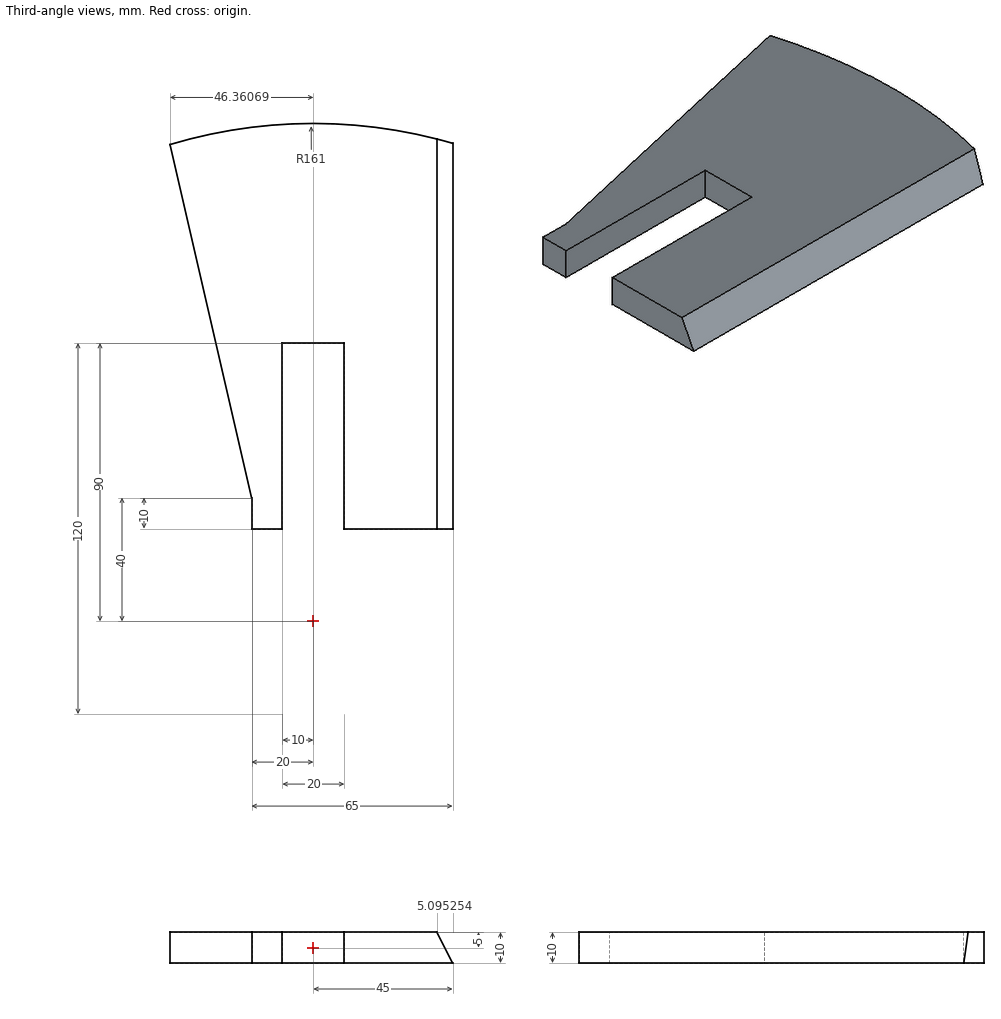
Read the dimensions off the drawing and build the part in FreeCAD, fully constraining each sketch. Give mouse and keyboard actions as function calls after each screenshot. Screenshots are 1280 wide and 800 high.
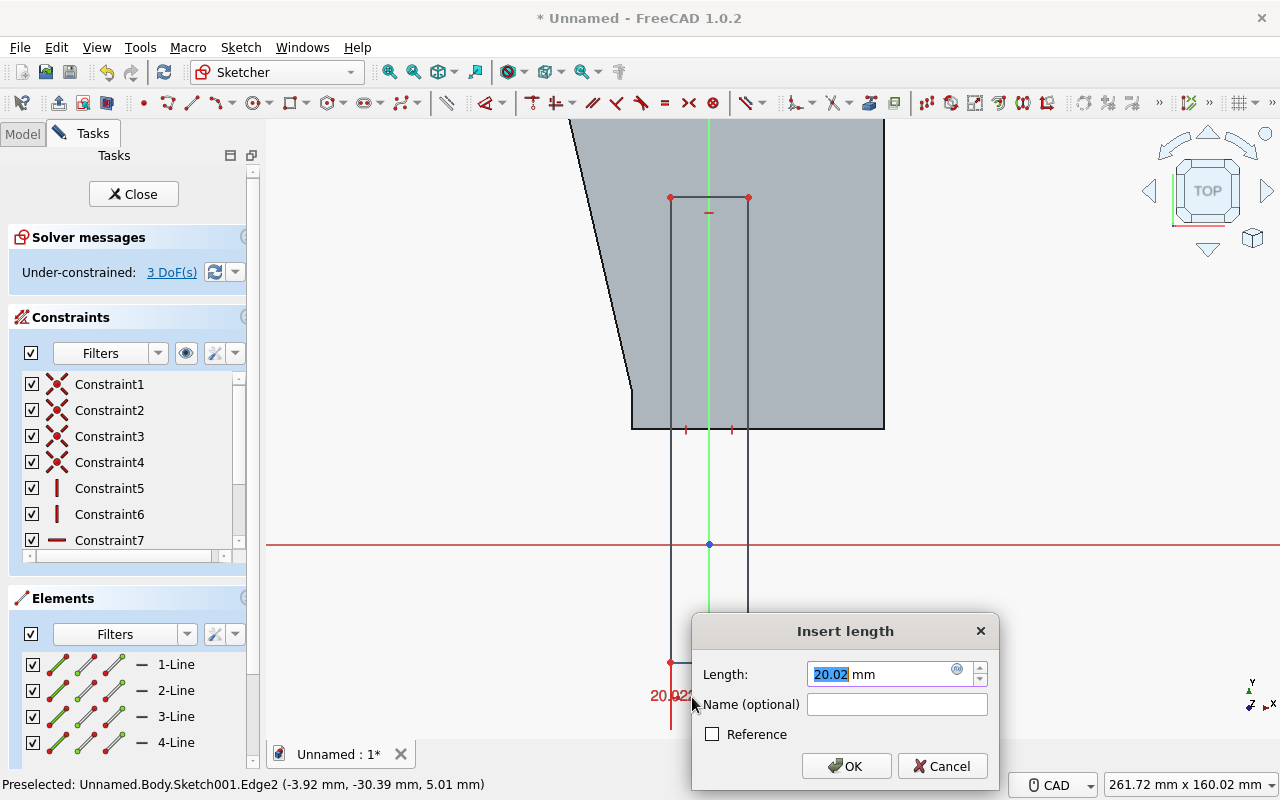
text(20)
key(Return)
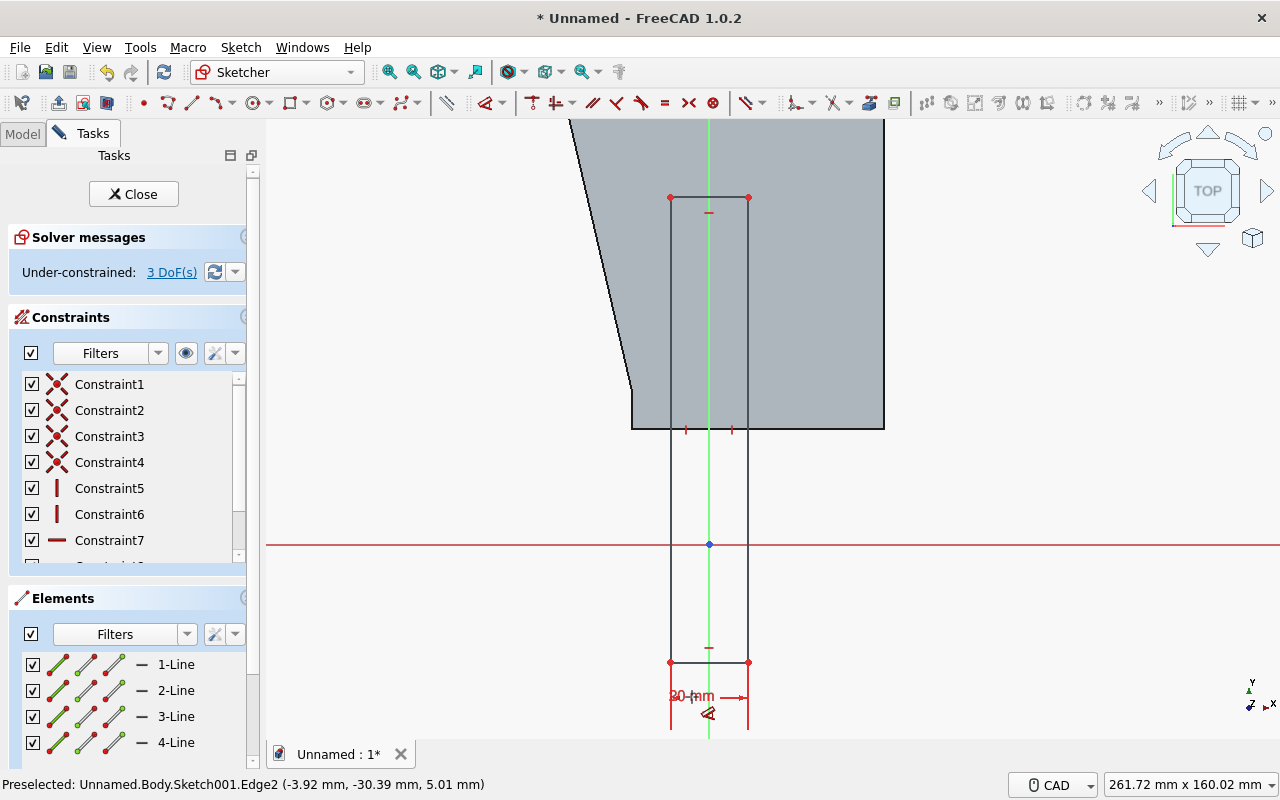
click(671, 337)
click(637, 430)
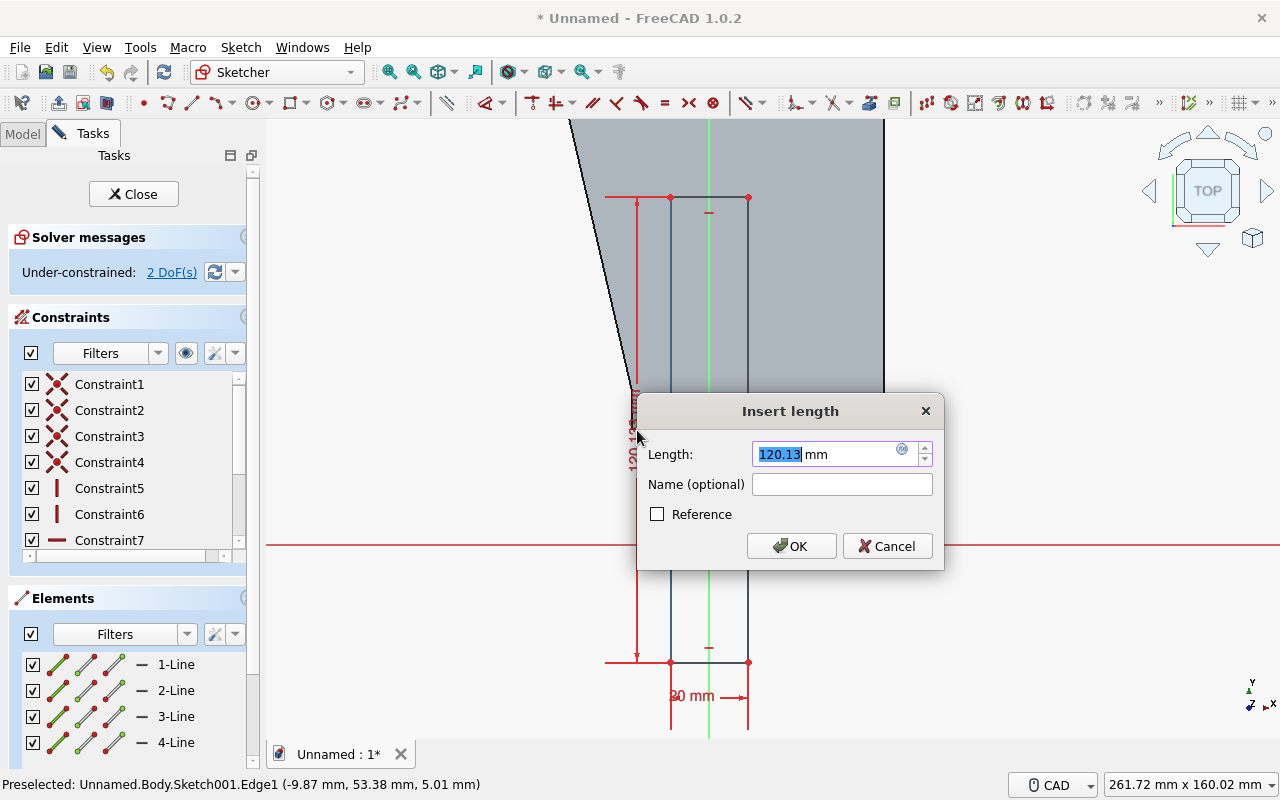
text(120)
key(Return)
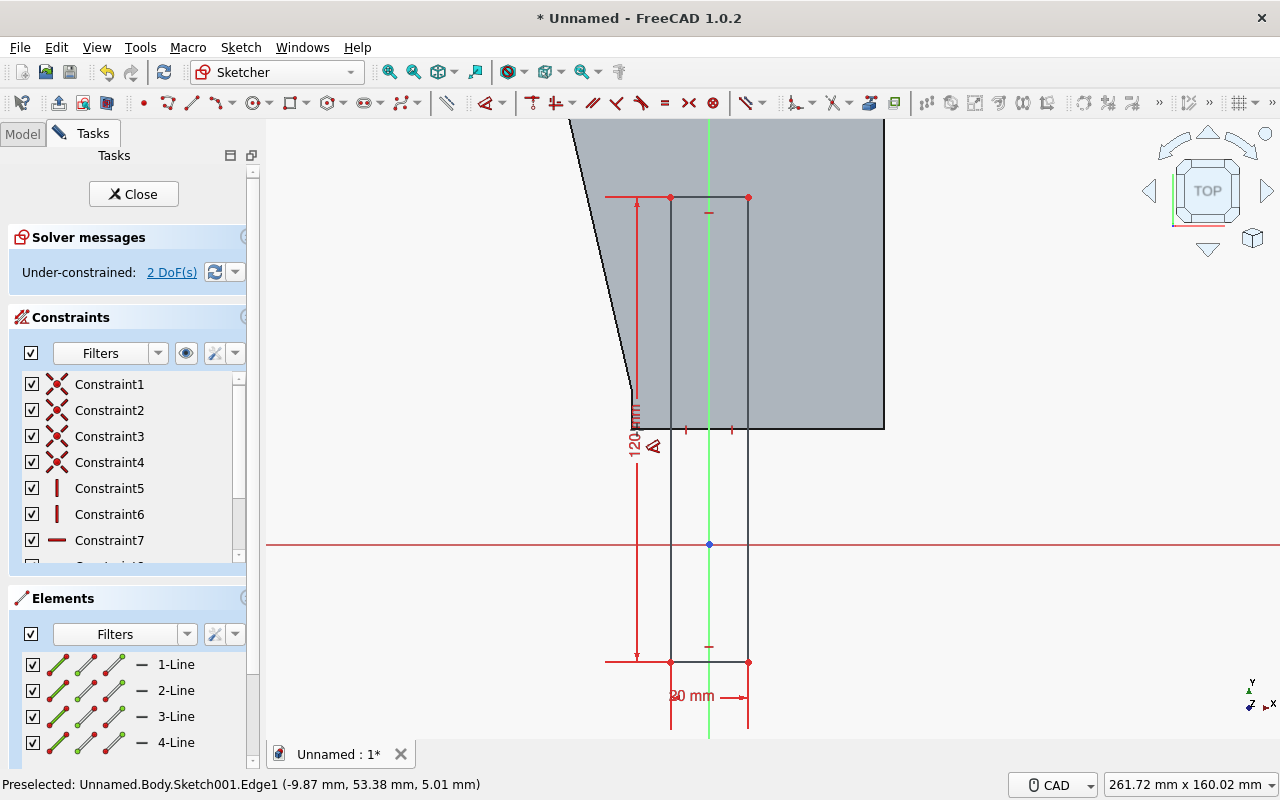
click(671, 197)
click(690, 163)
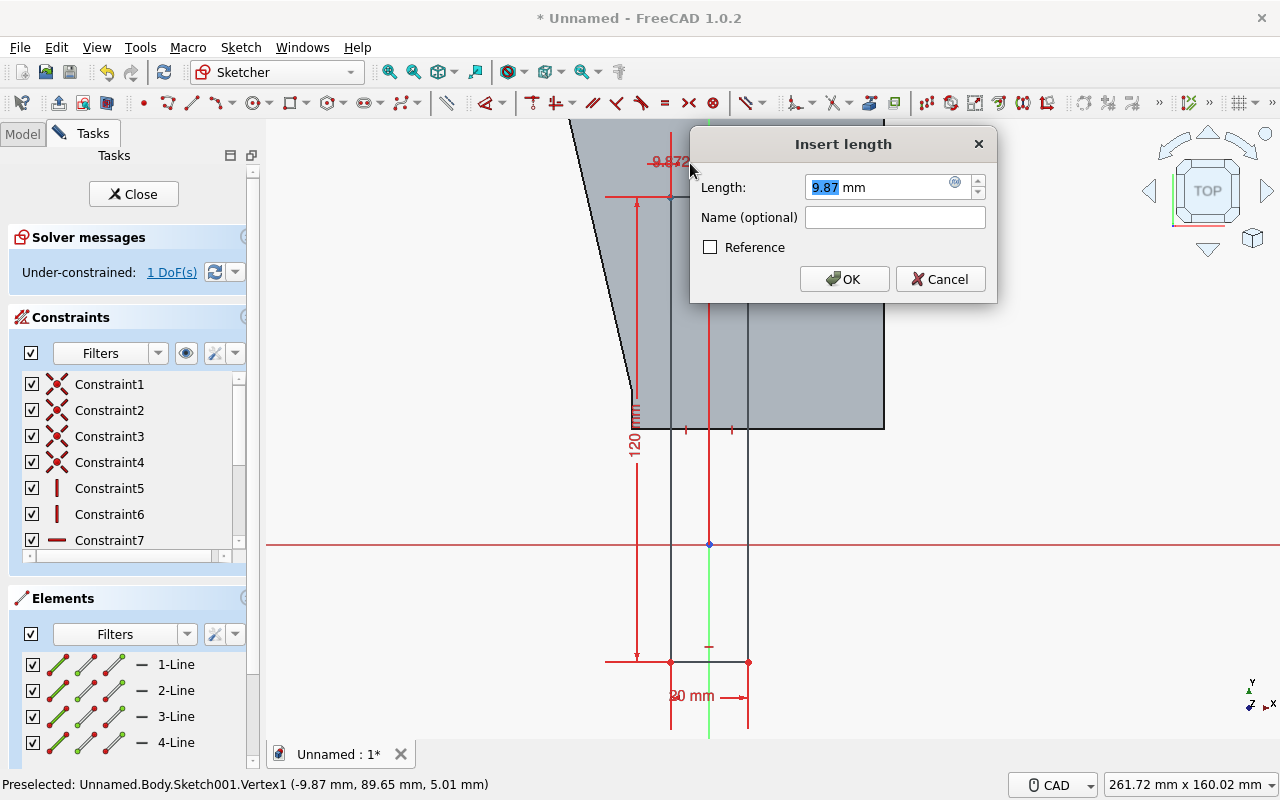
text(10)
key(Return)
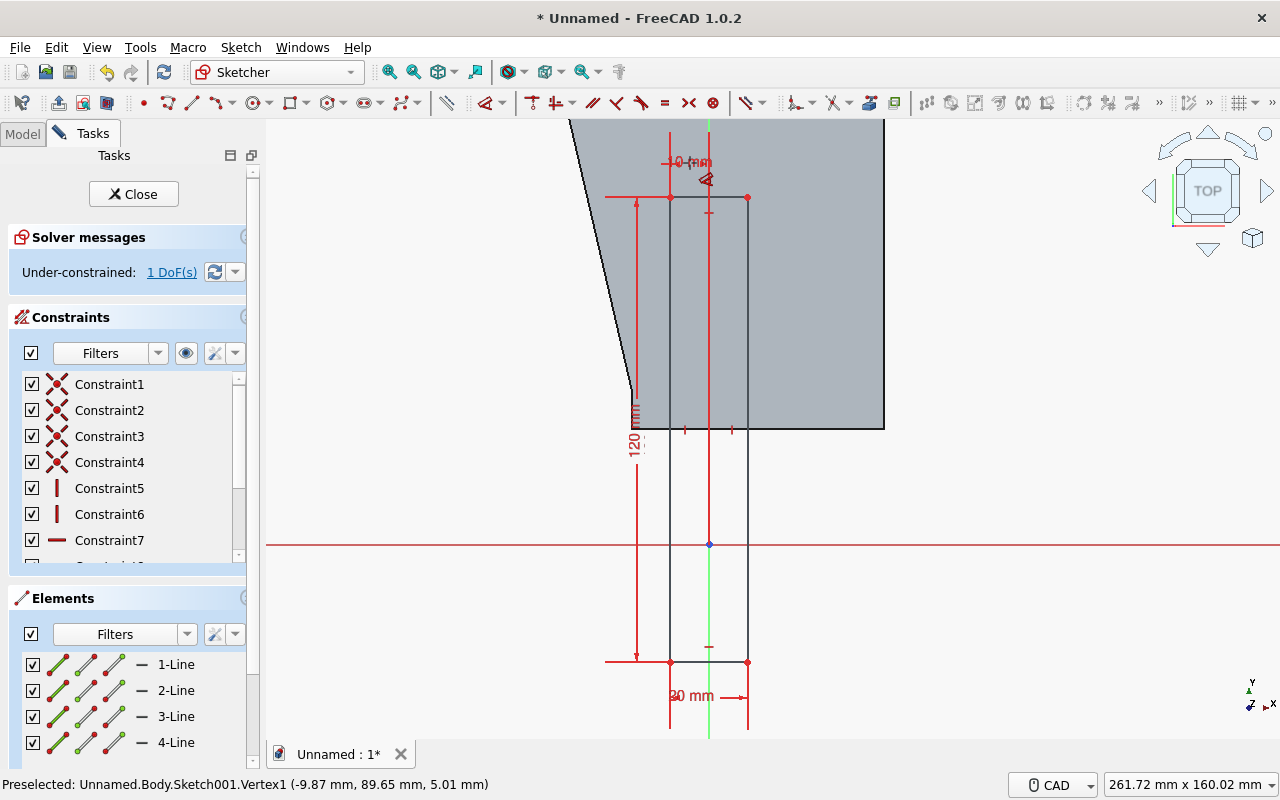
click(670, 197)
click(636, 371)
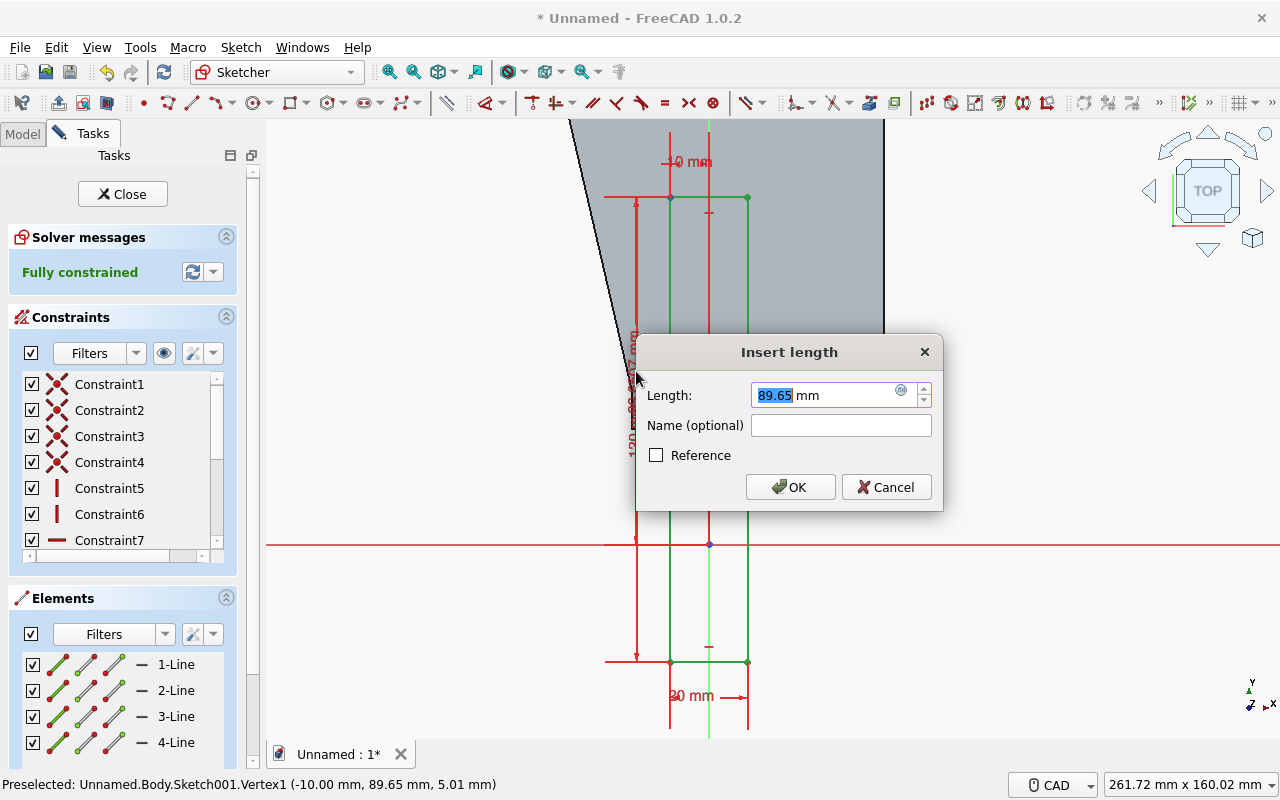
text(90)
key(Return)
key(Escape)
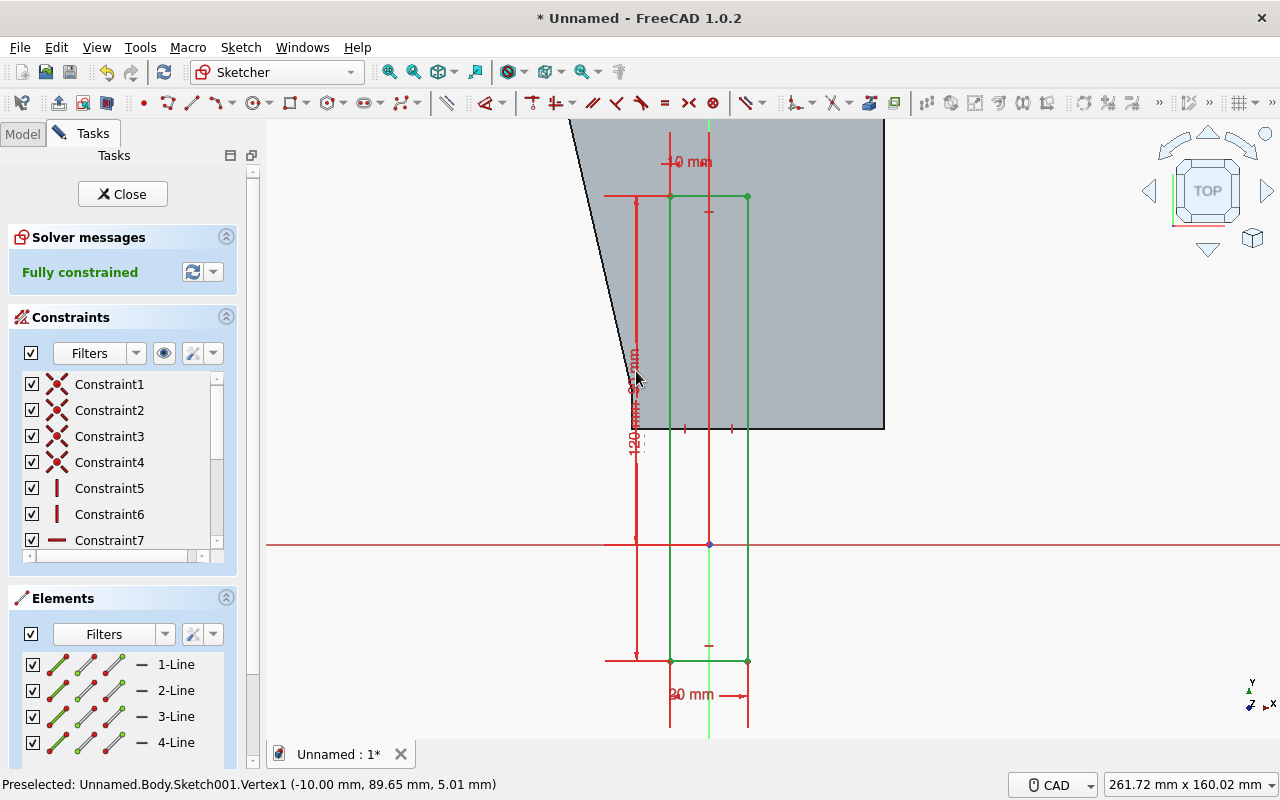
click(123, 194)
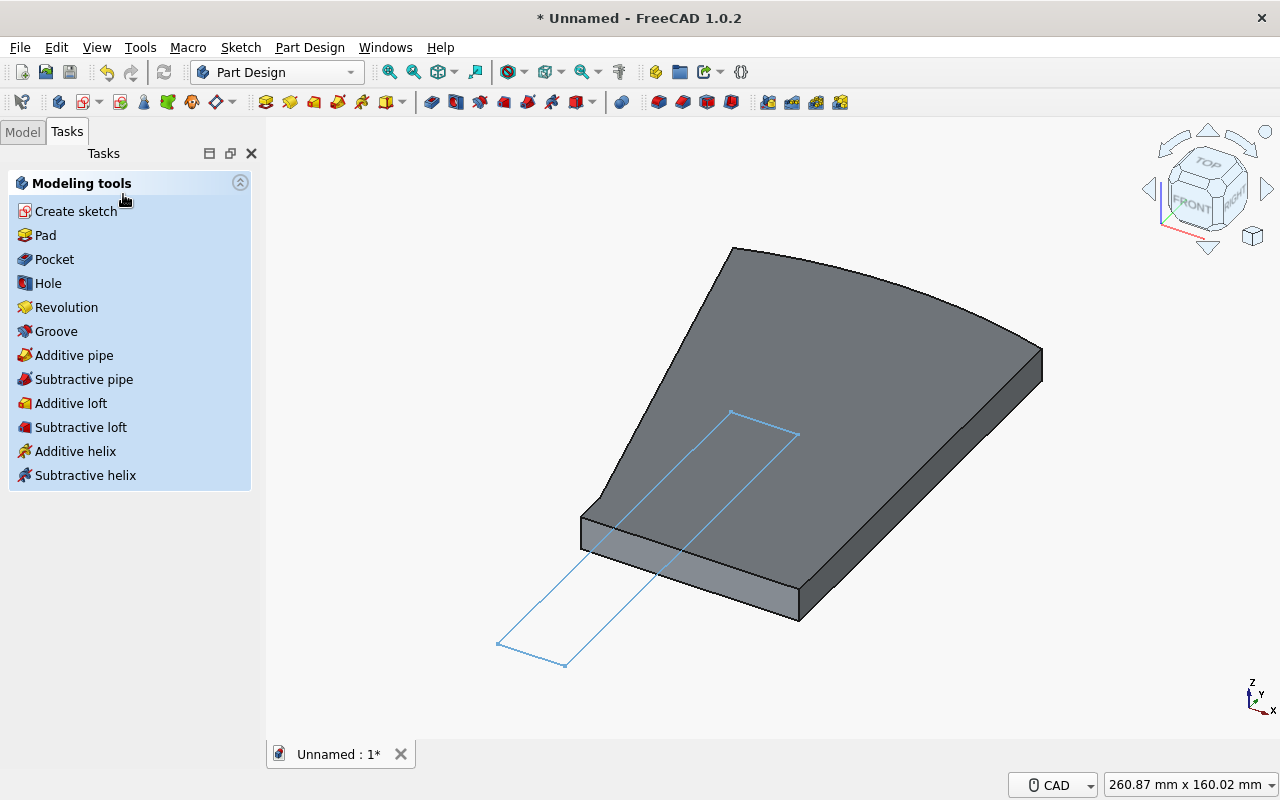
click(432, 102)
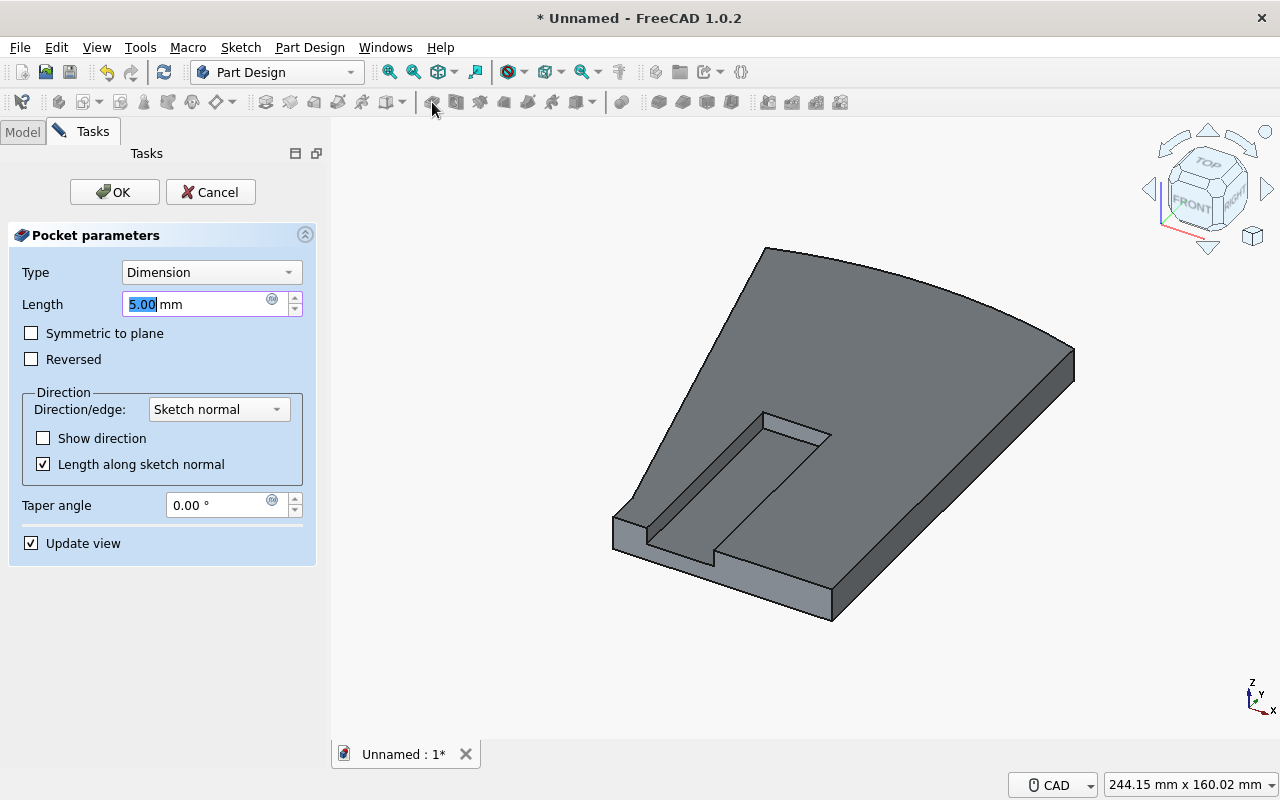
text(10)
key(Tab)